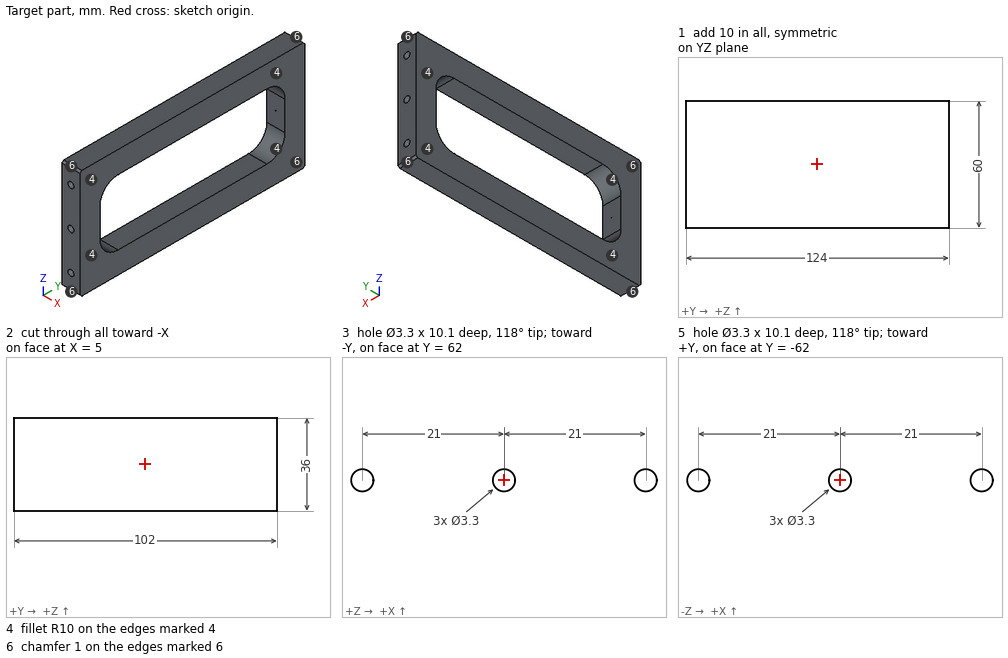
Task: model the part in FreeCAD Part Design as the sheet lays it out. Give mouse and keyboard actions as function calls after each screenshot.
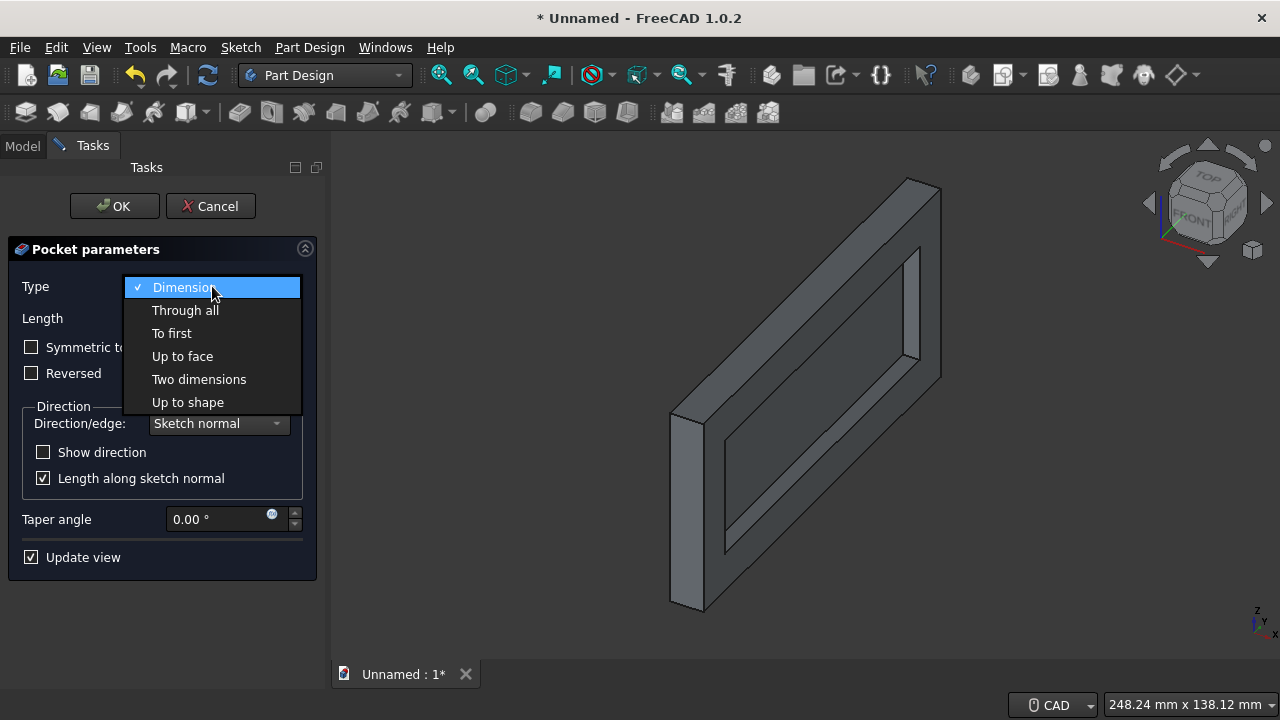
click(212, 310)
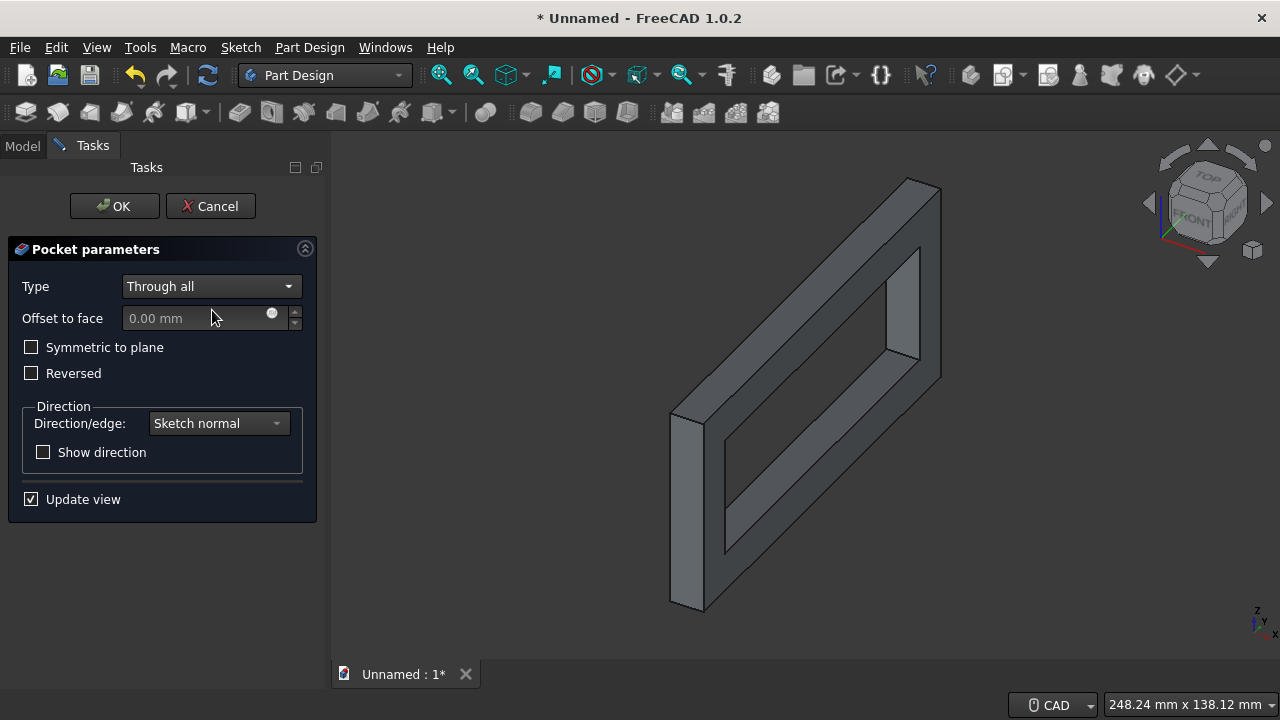
click(115, 206)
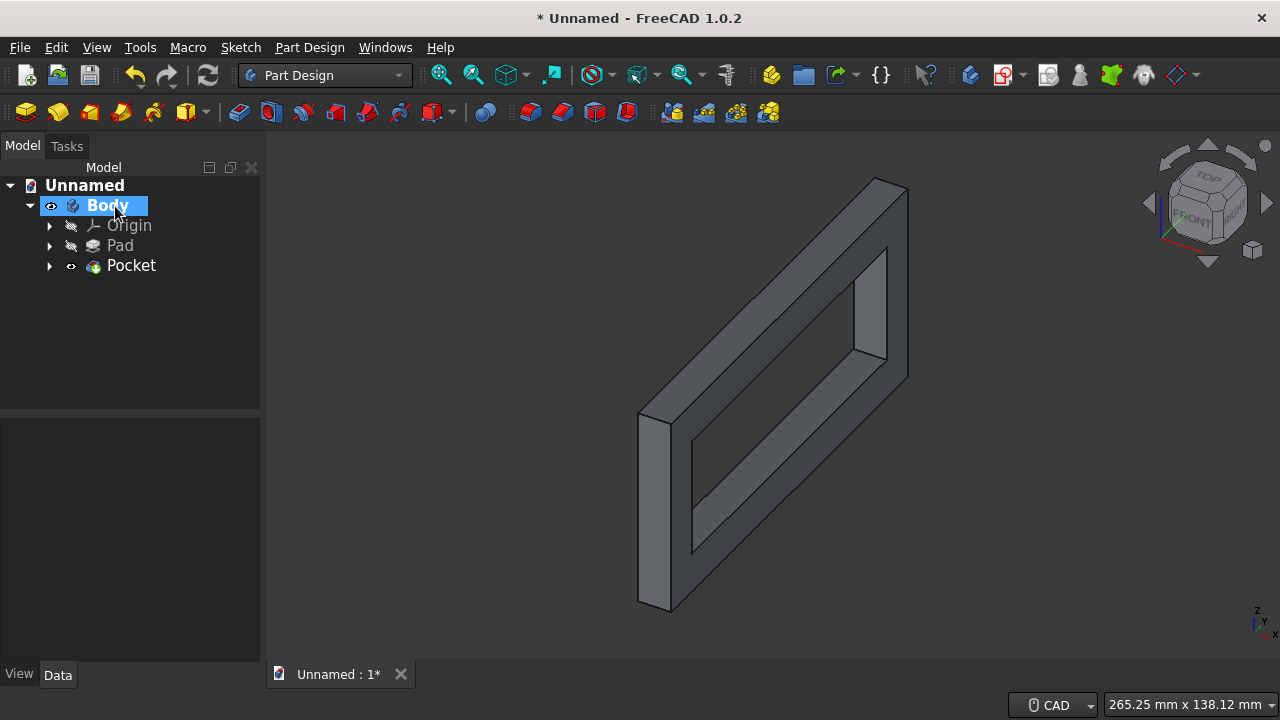
key(4)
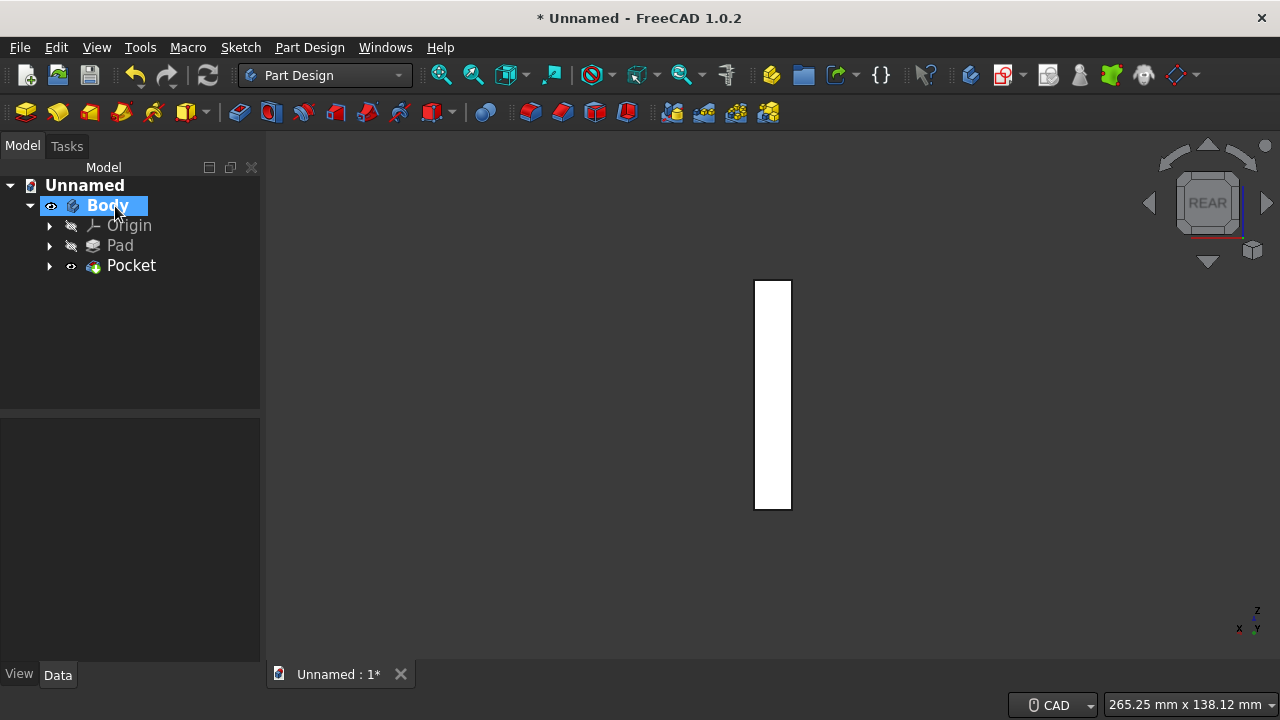
click(442, 76)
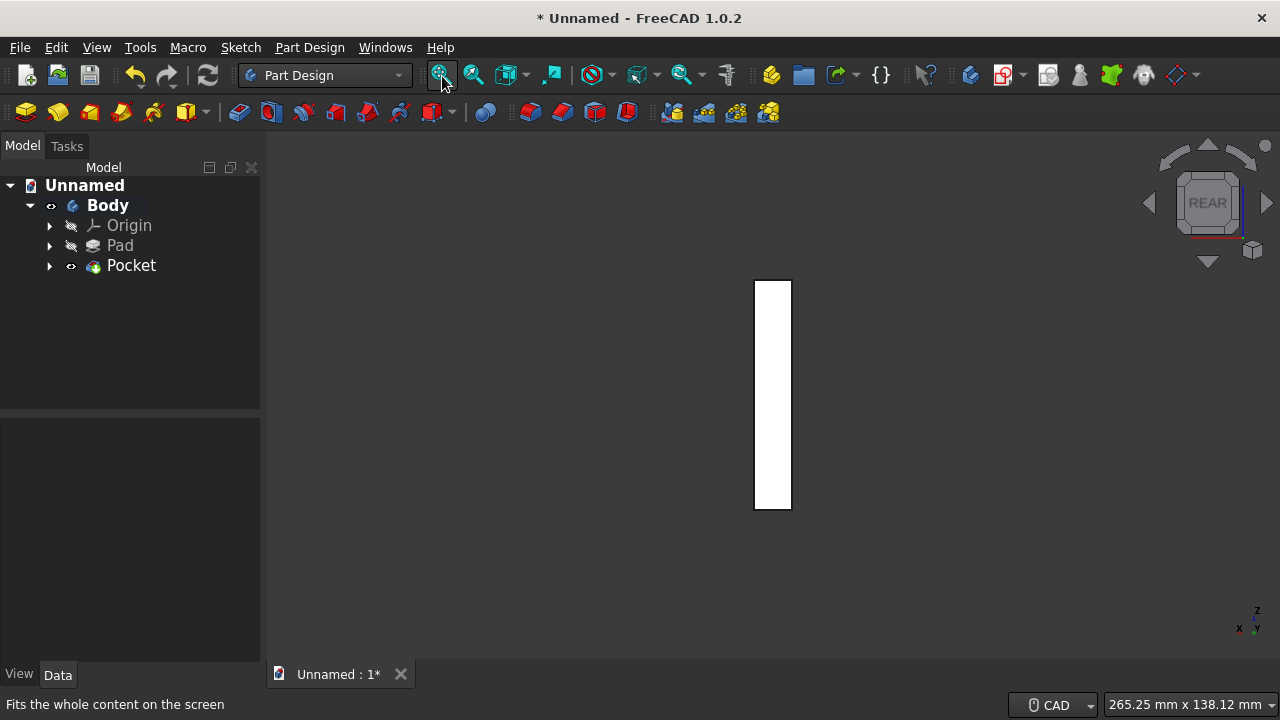
click(773, 427)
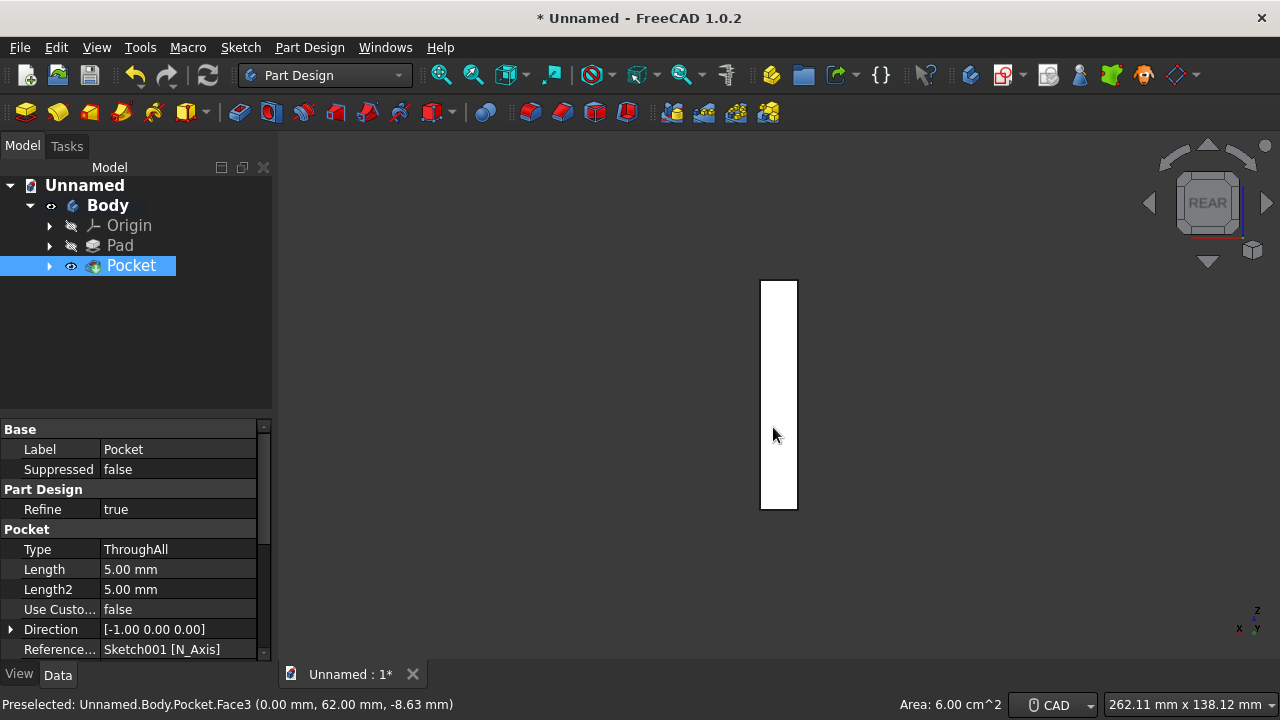
click(1004, 76)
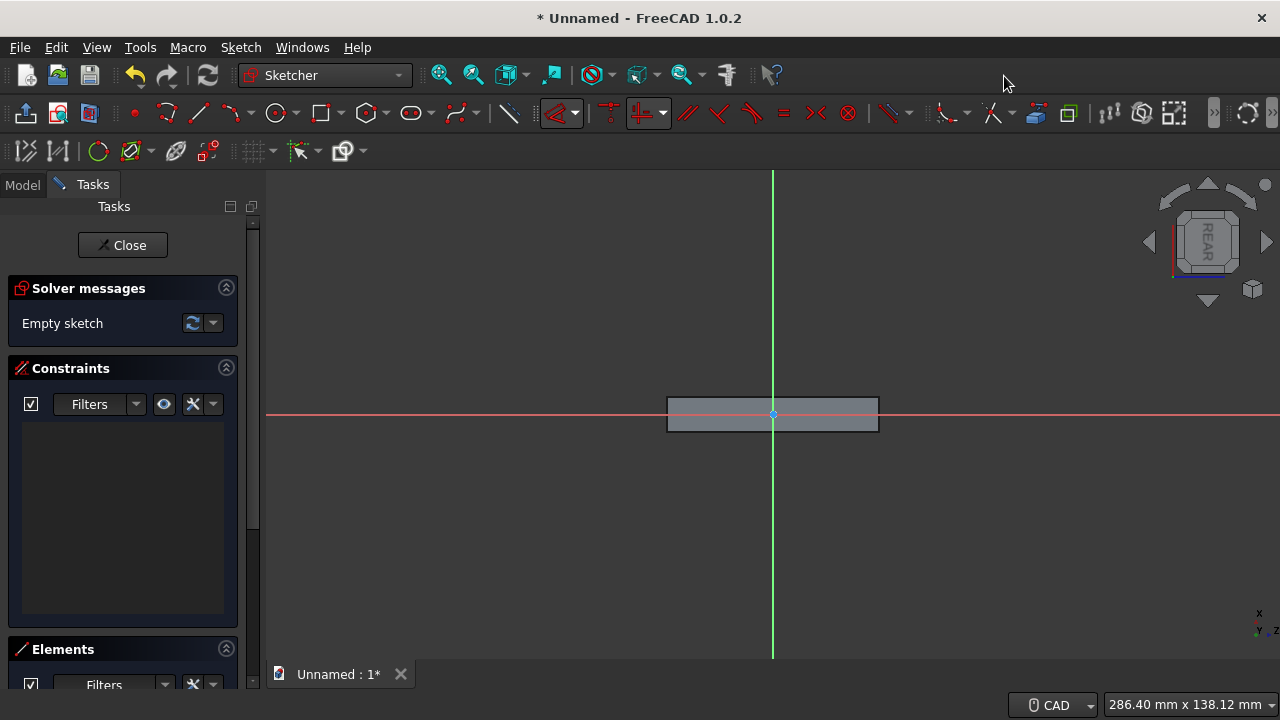
scroll(803, 414, up, 6)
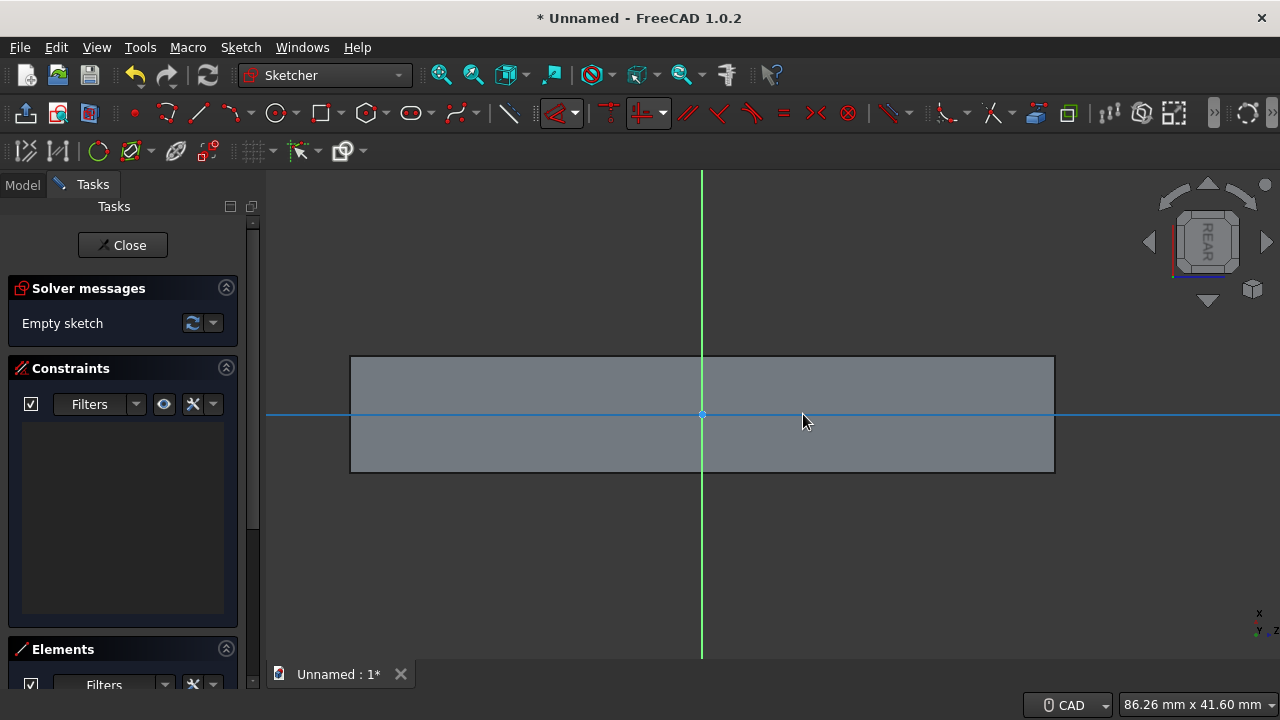
click(276, 114)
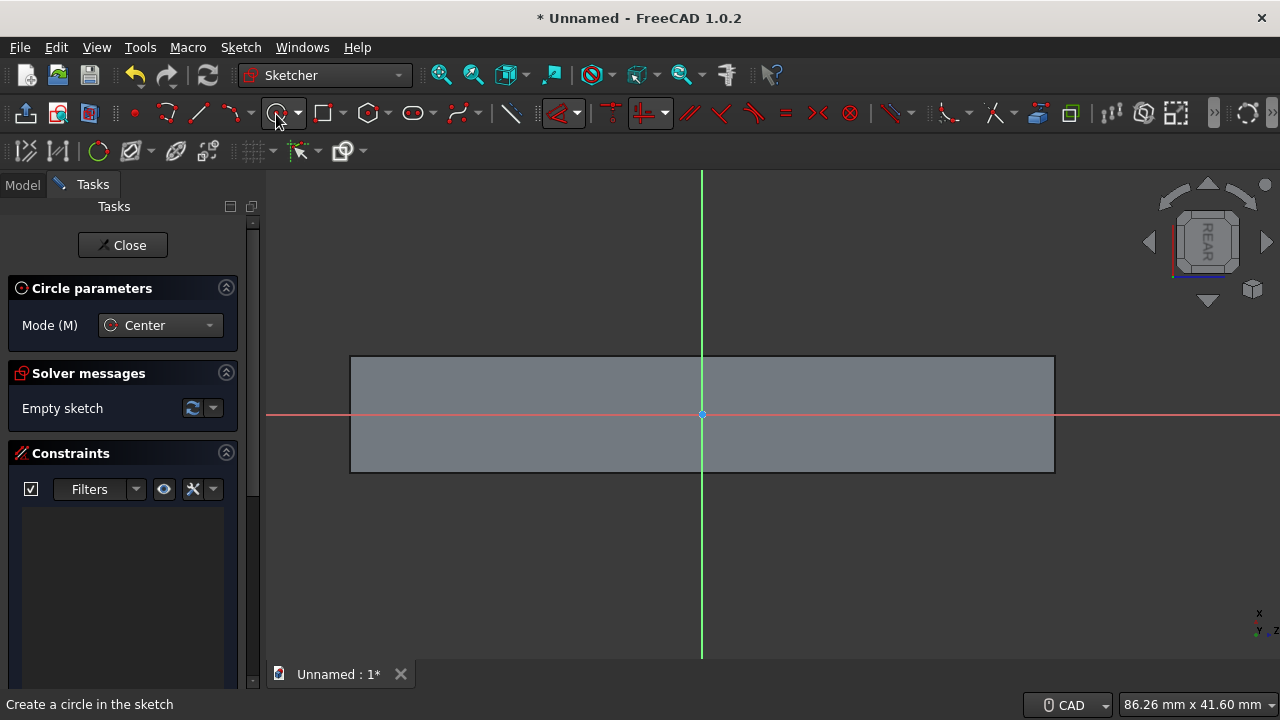
click(702, 414)
move(716, 401)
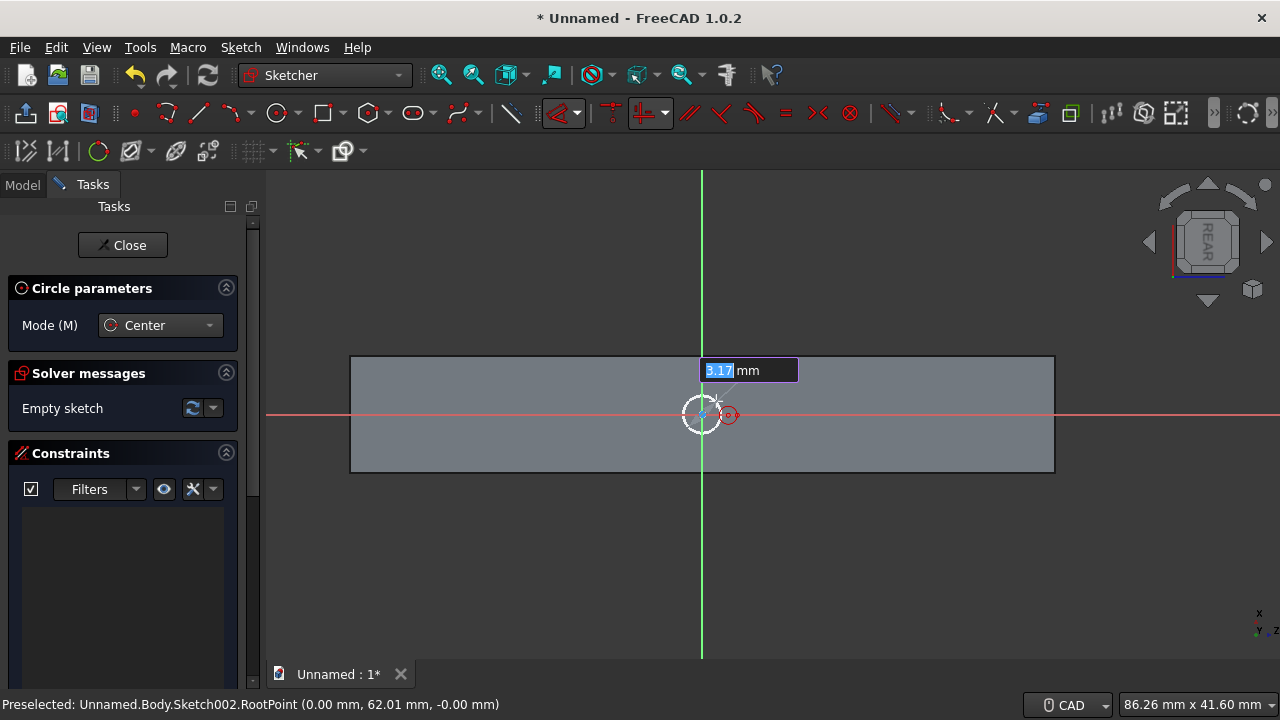
text(3.3)
key(Return)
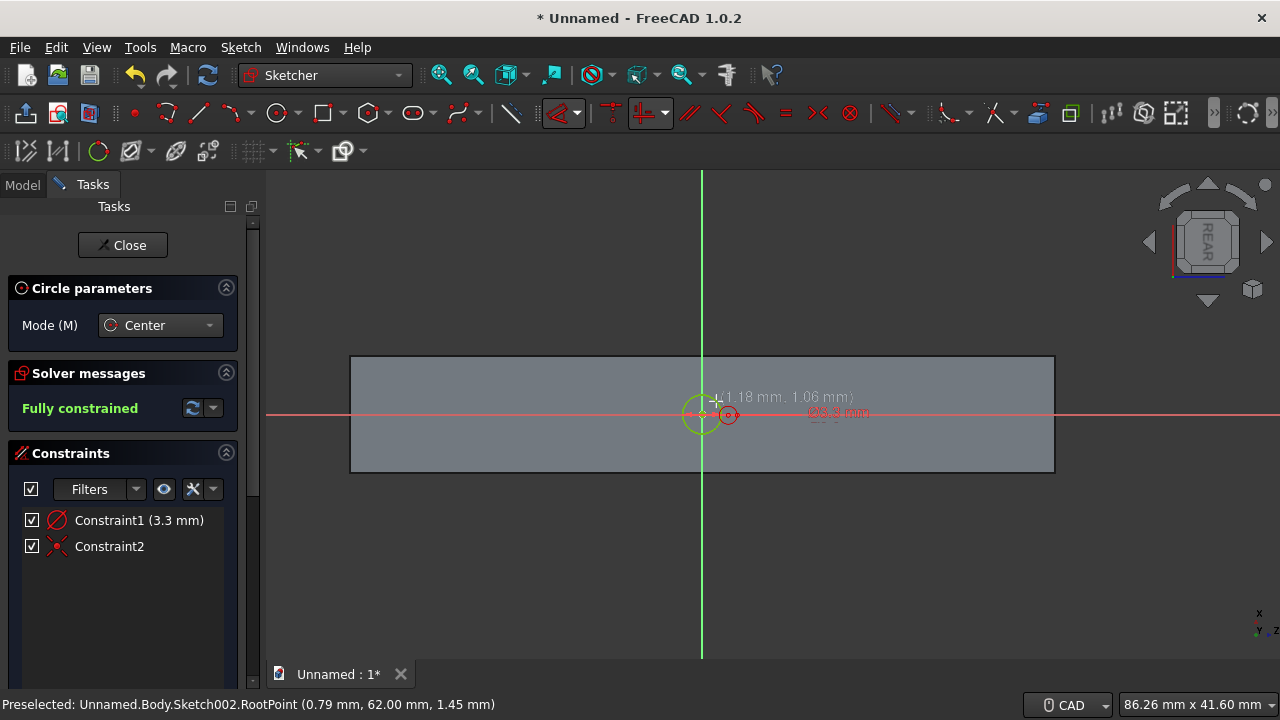
click(455, 414)
move(462, 396)